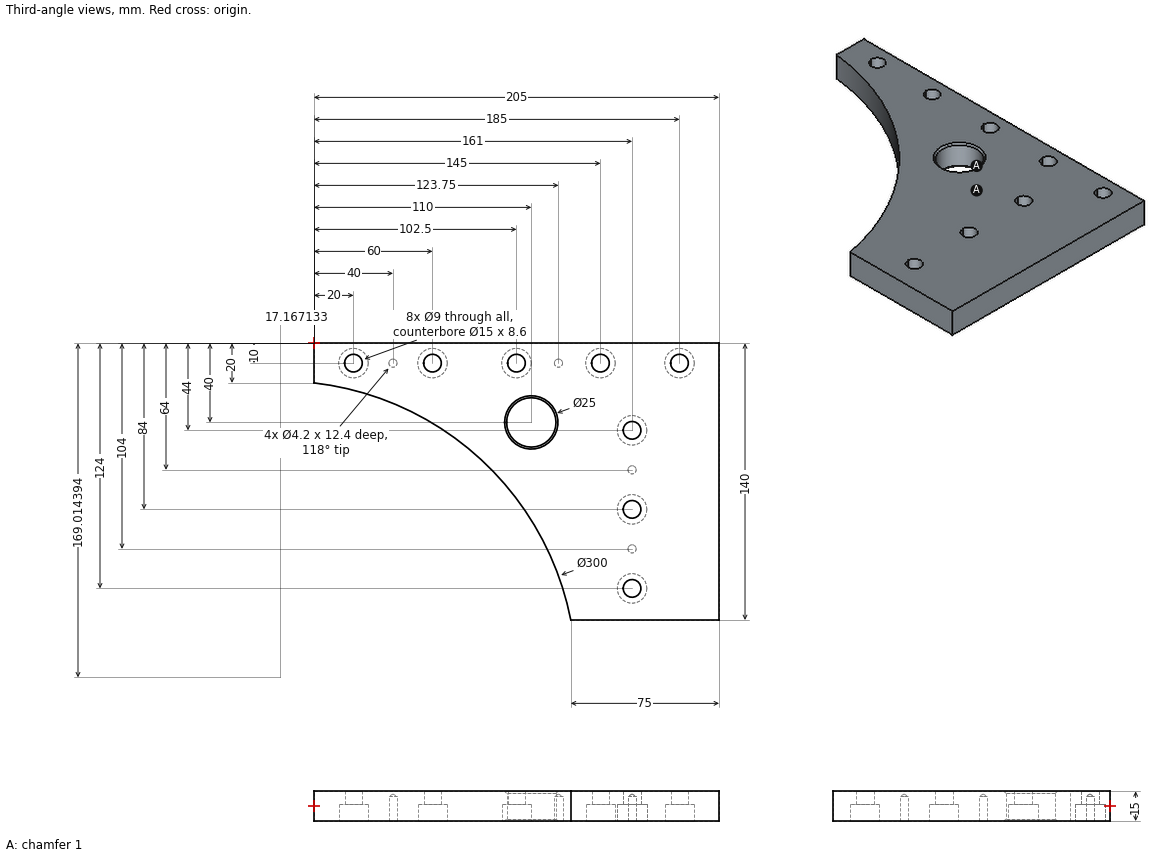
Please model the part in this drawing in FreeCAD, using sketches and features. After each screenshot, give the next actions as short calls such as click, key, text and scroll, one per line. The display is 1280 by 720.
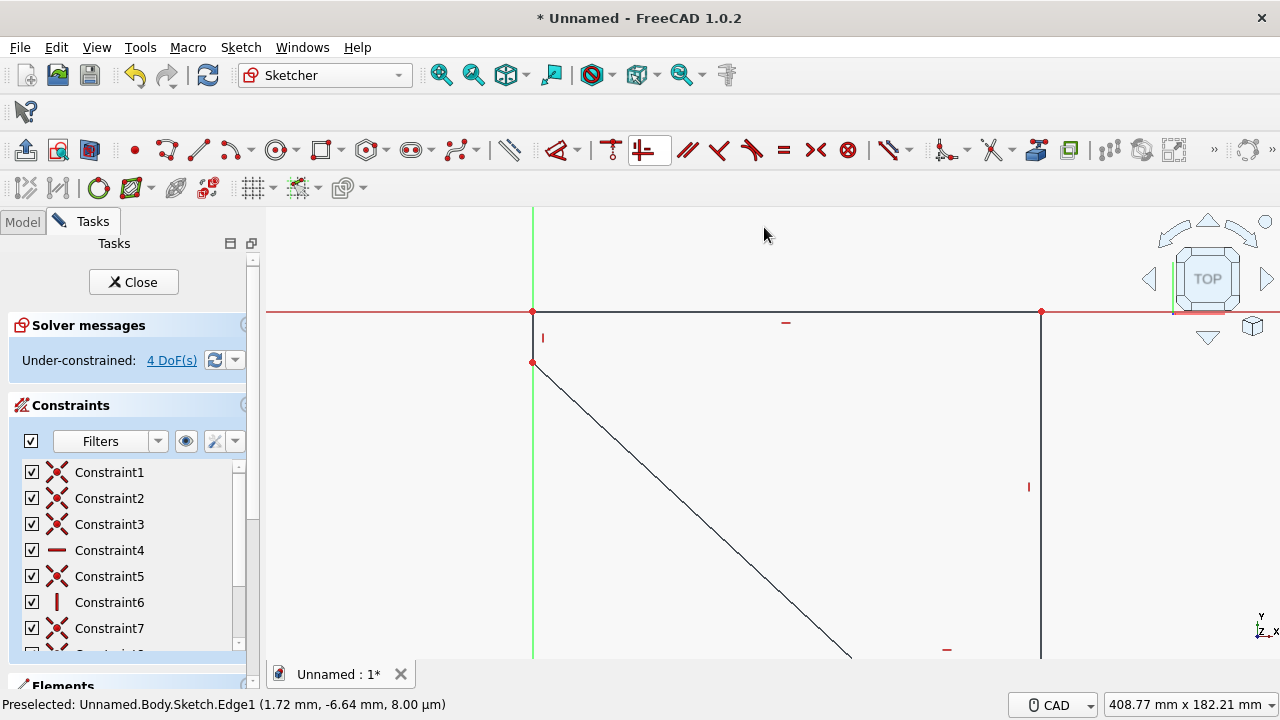
click(533, 327)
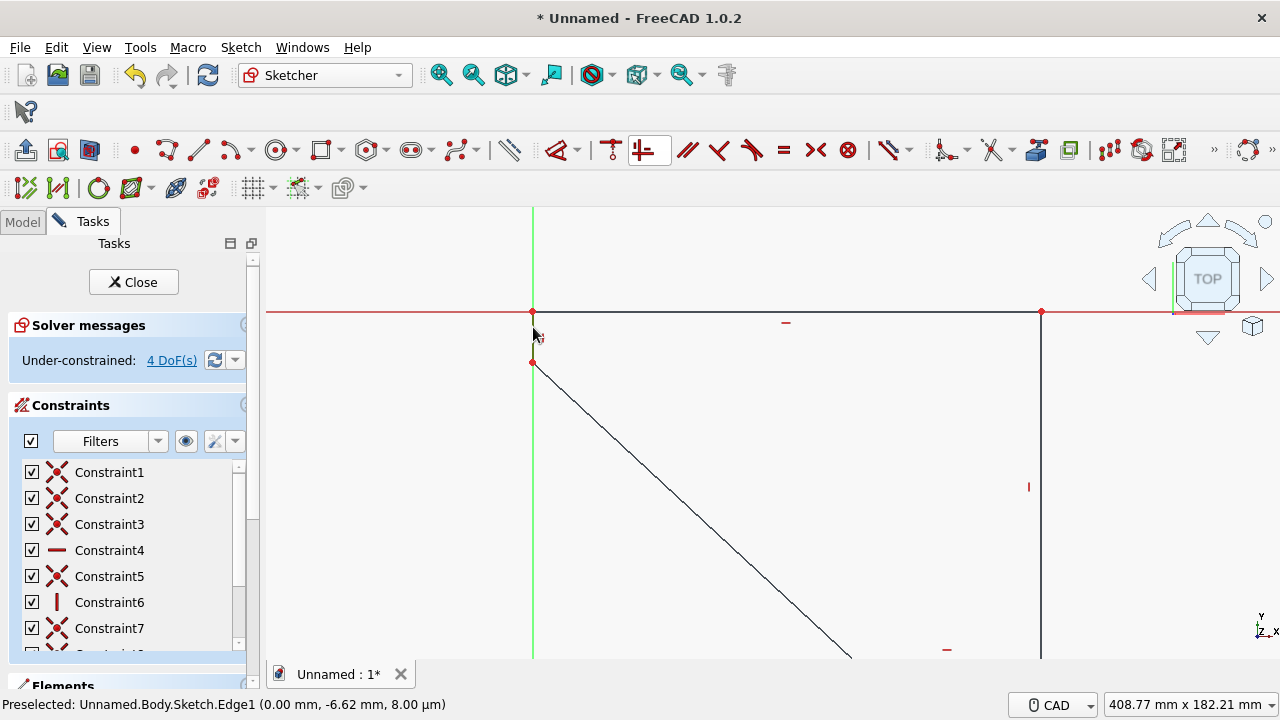
click(580, 150)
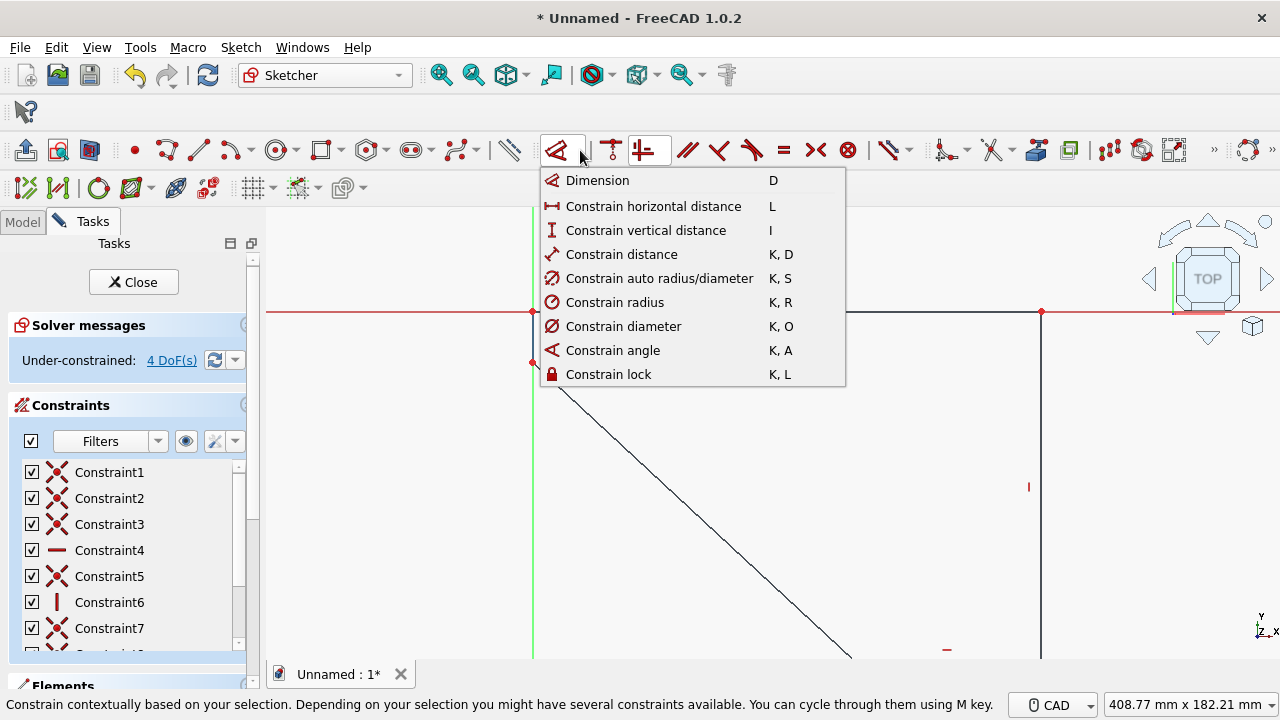
click(693, 230)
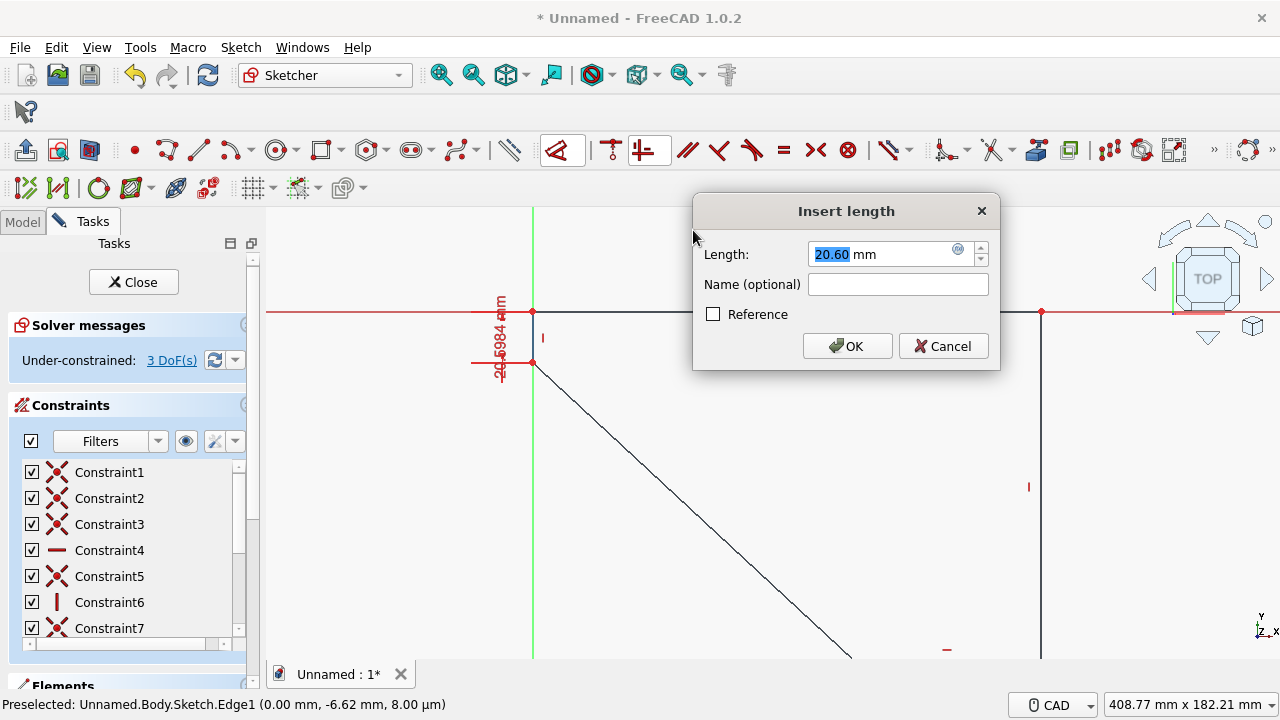
text(20)
key(Return)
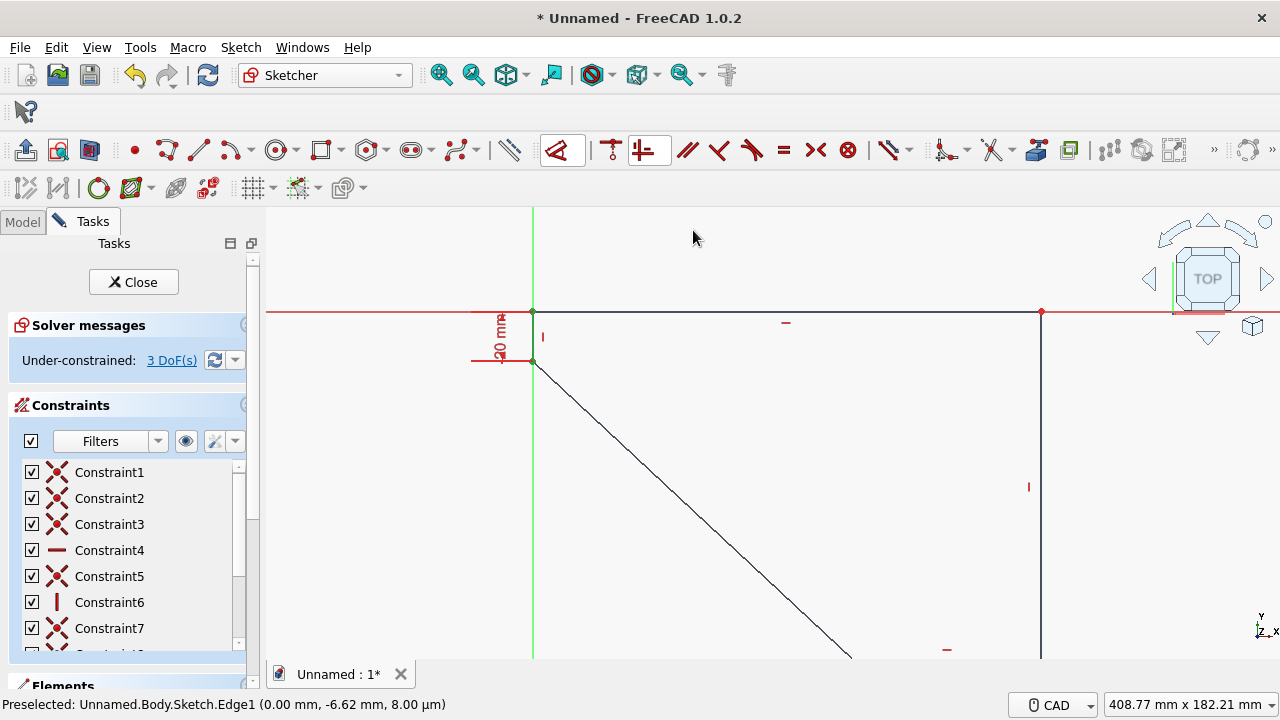
scroll(332, 235, down, 1)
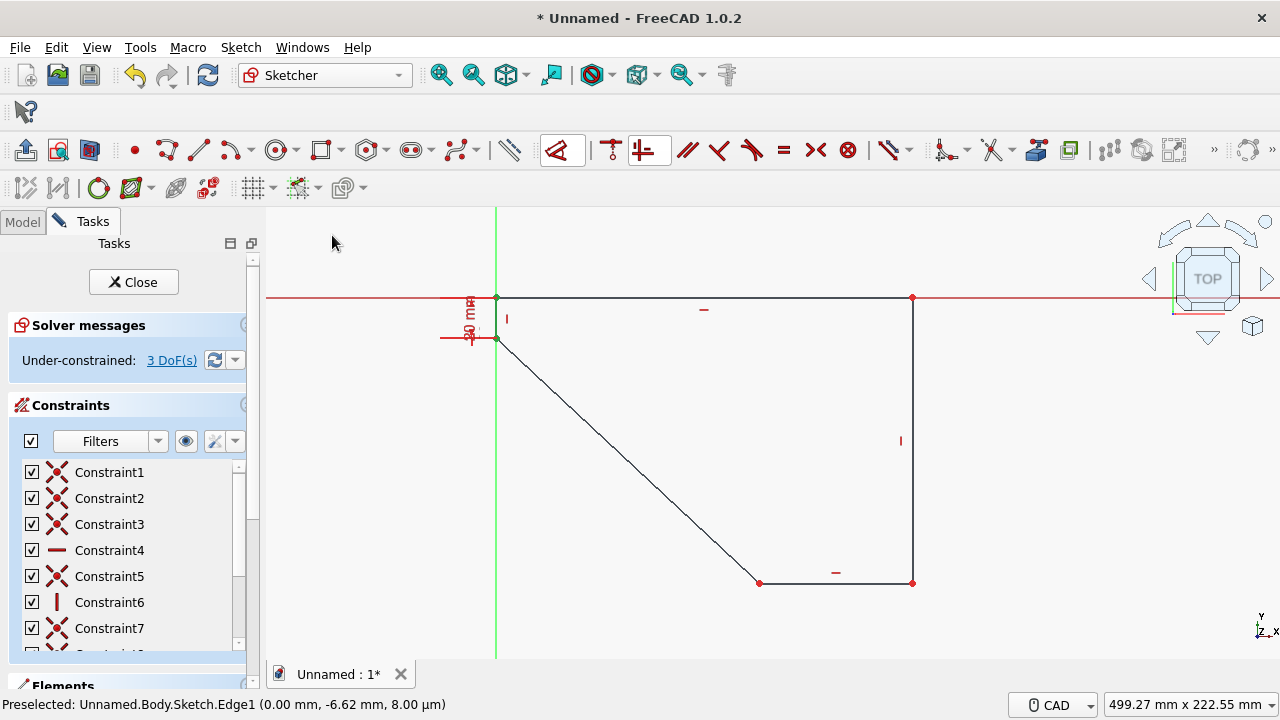
click(806, 584)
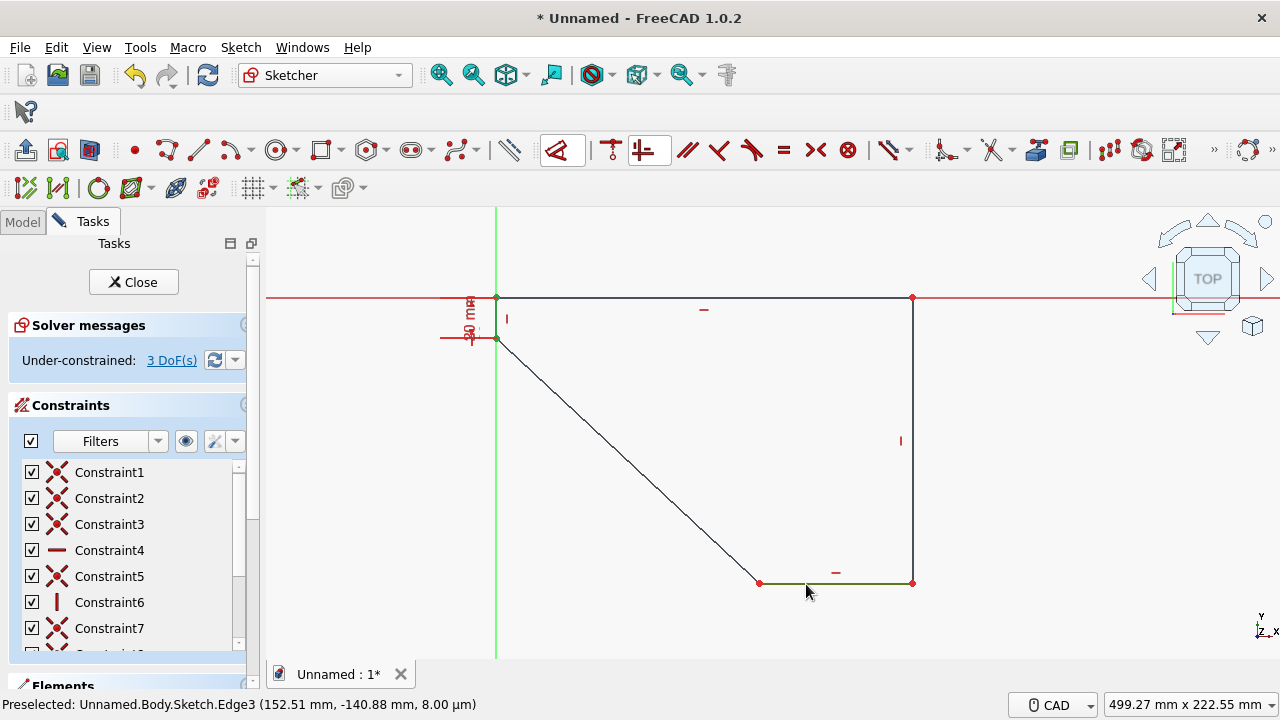
click(580, 150)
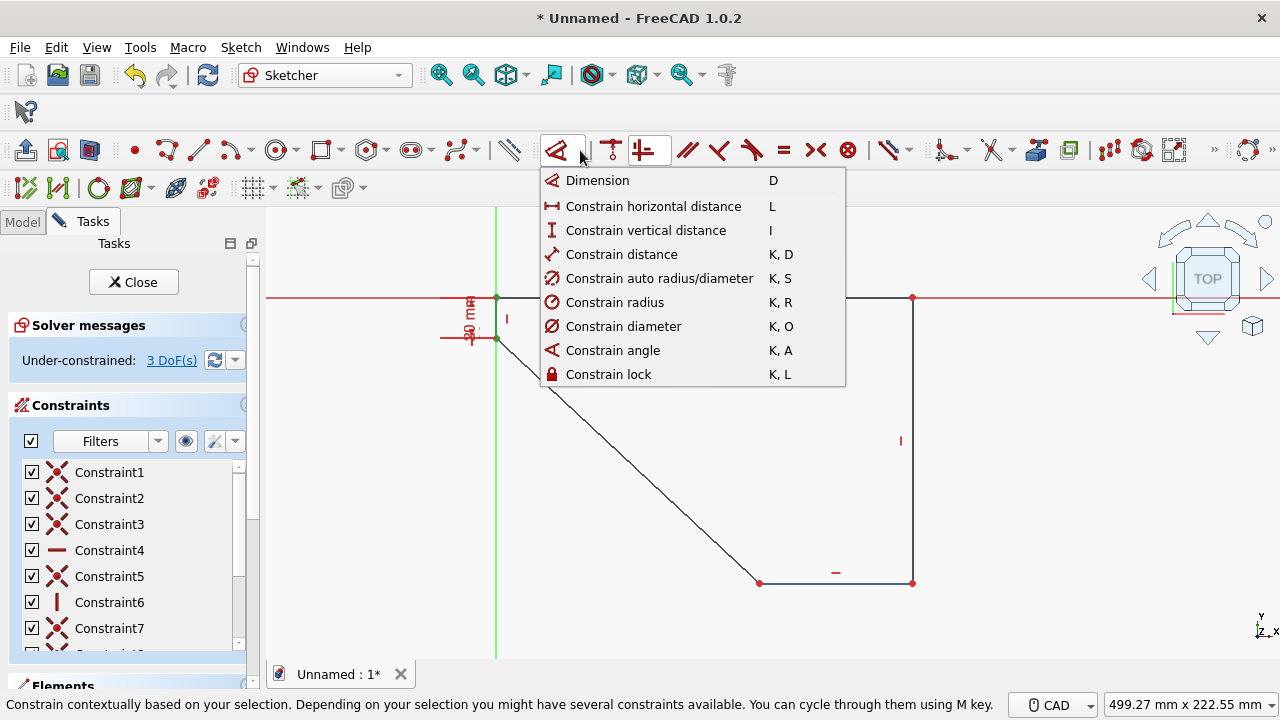
click(693, 206)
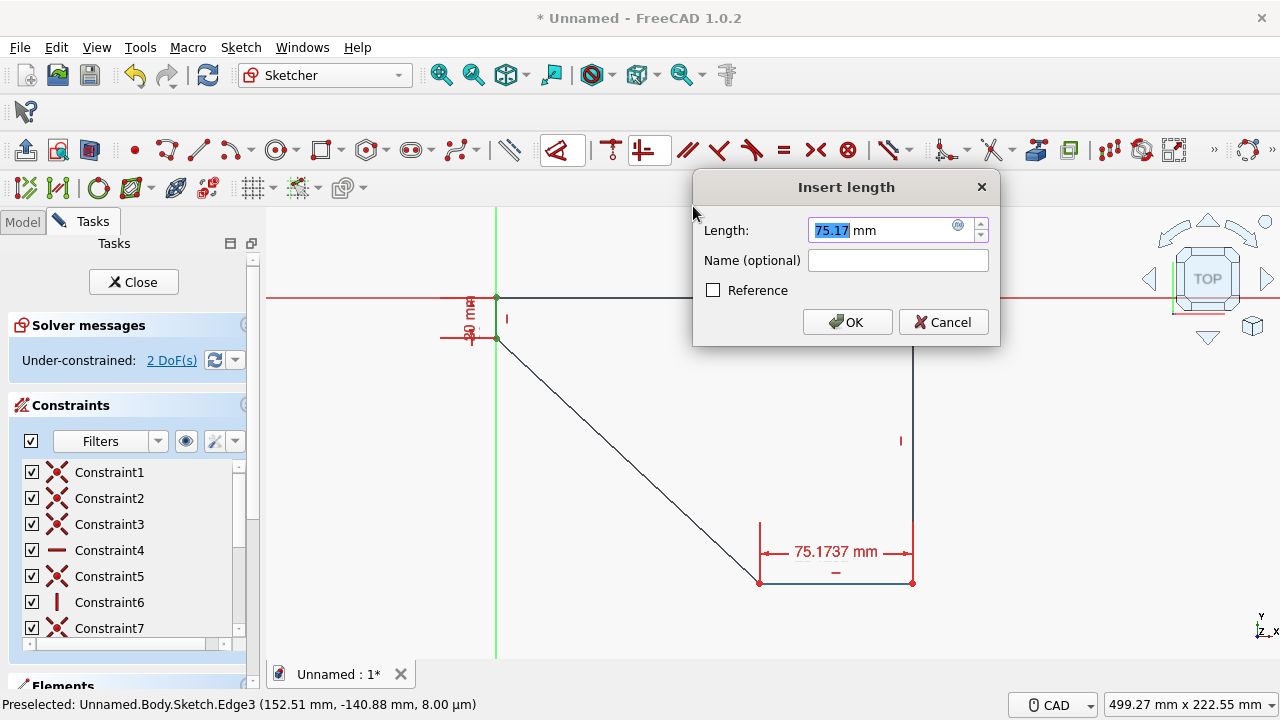
text(75)
key(Return)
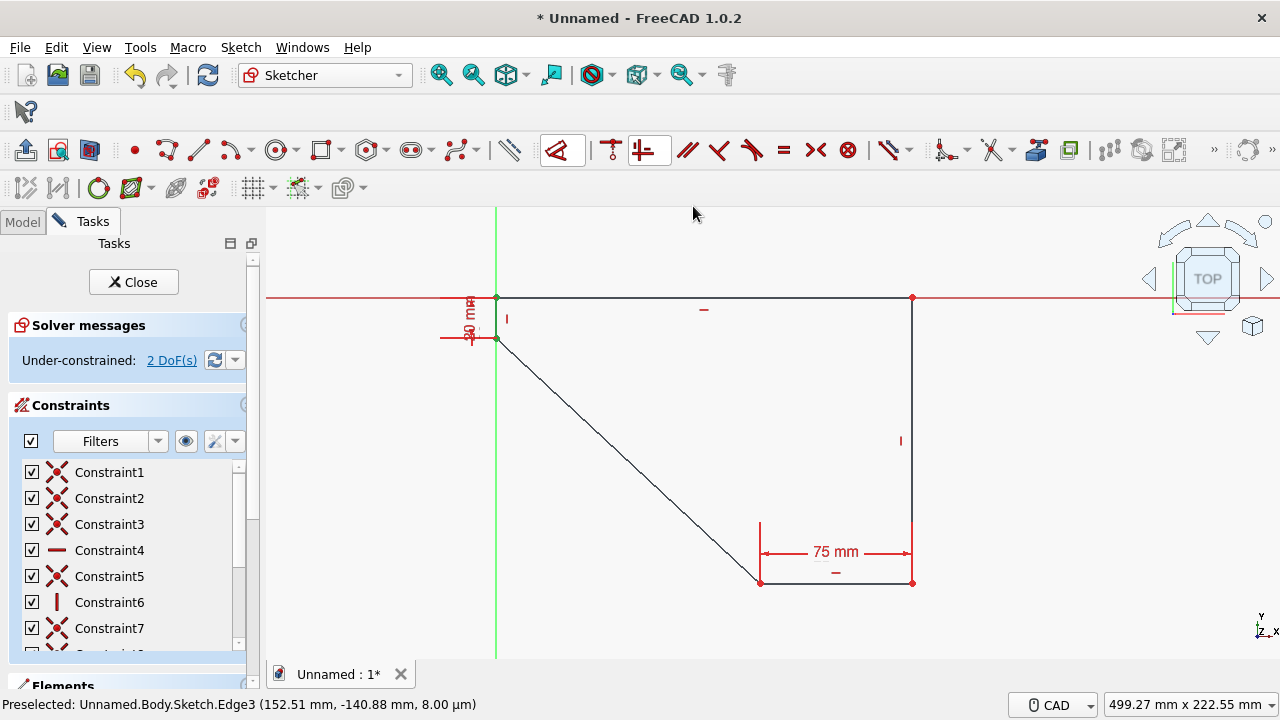
click(912, 498)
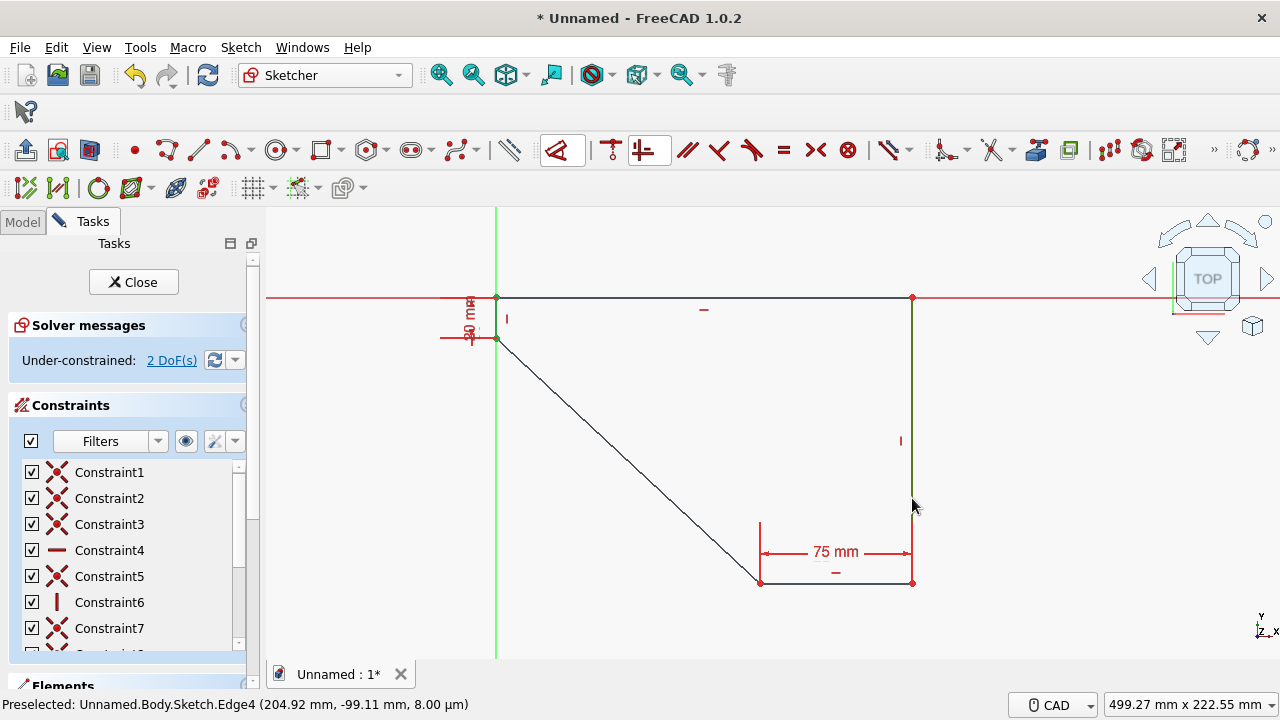
click(580, 150)